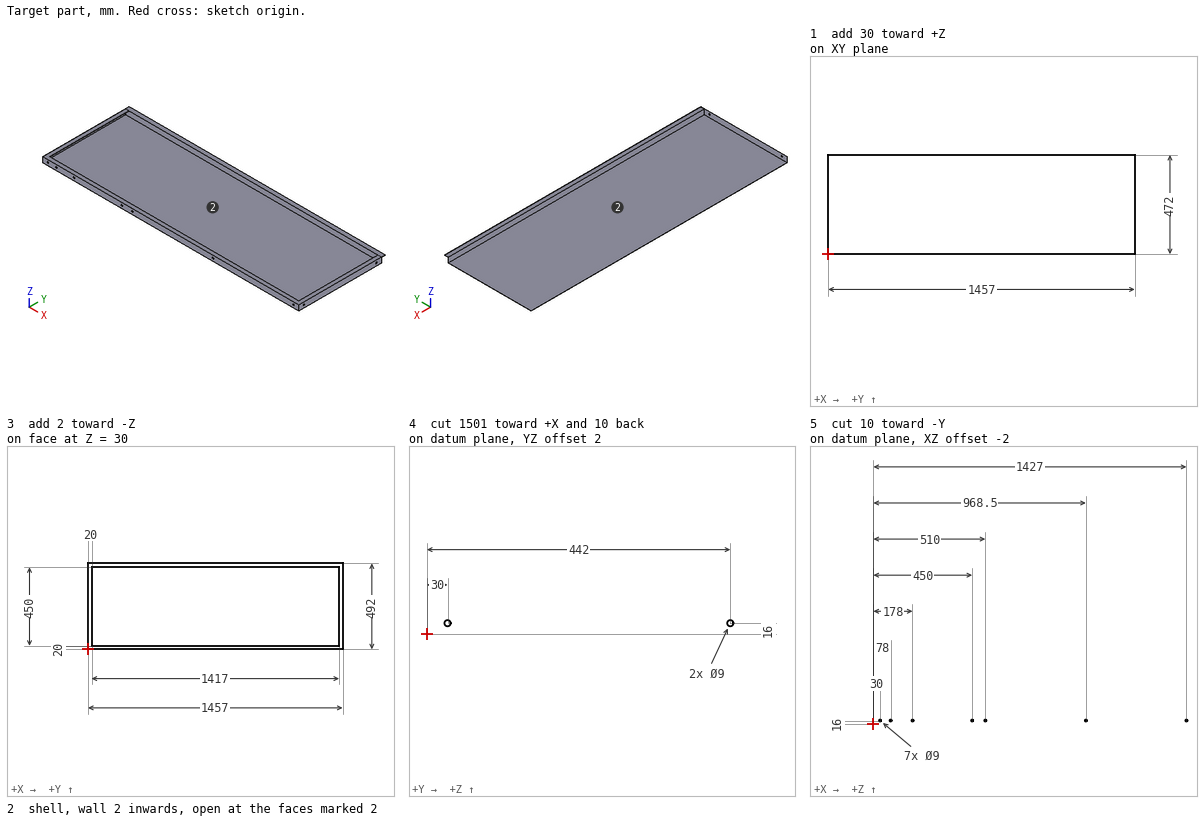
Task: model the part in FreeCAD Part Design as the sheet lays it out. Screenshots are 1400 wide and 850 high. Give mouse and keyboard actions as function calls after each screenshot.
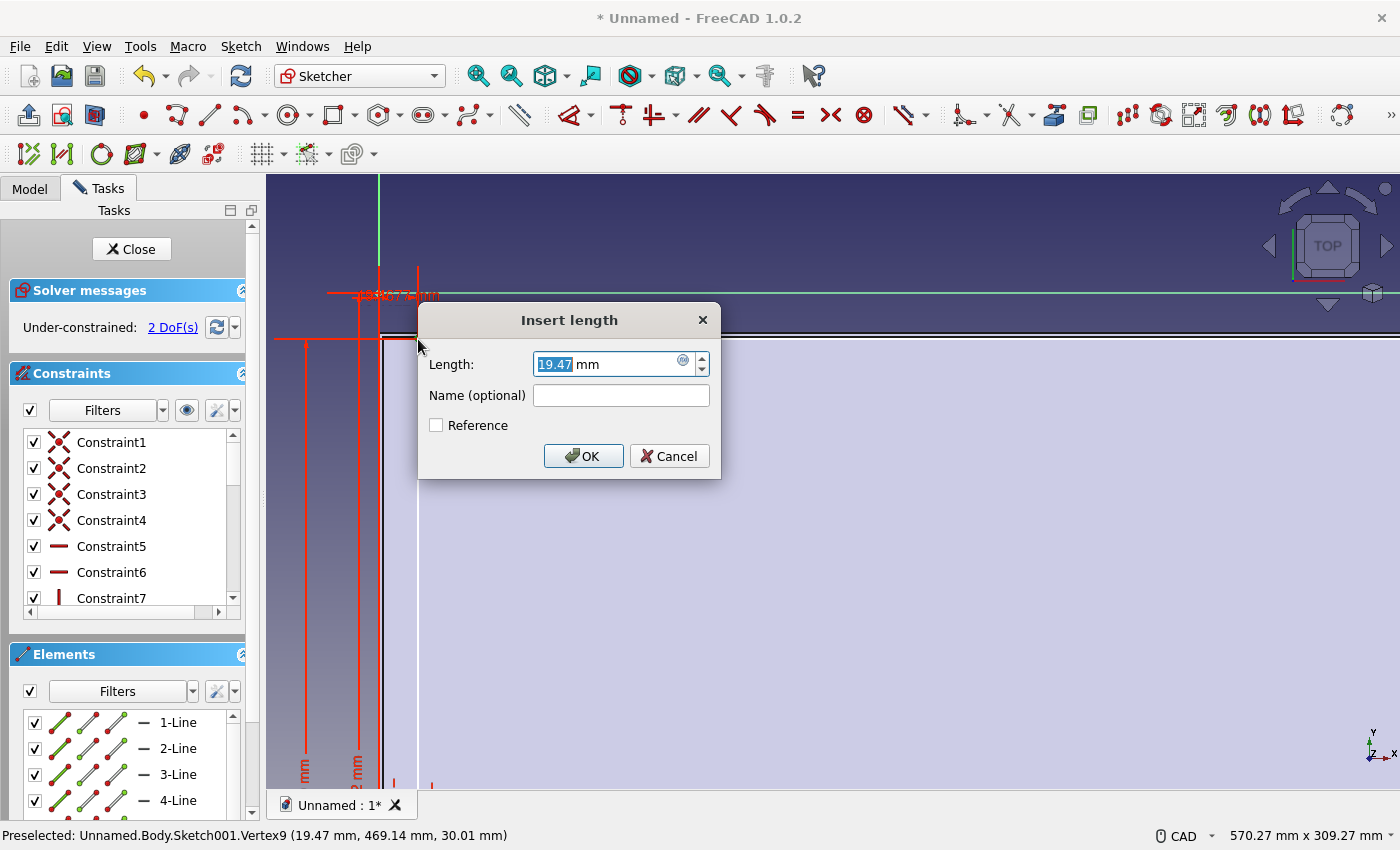
text(20)
key(Return)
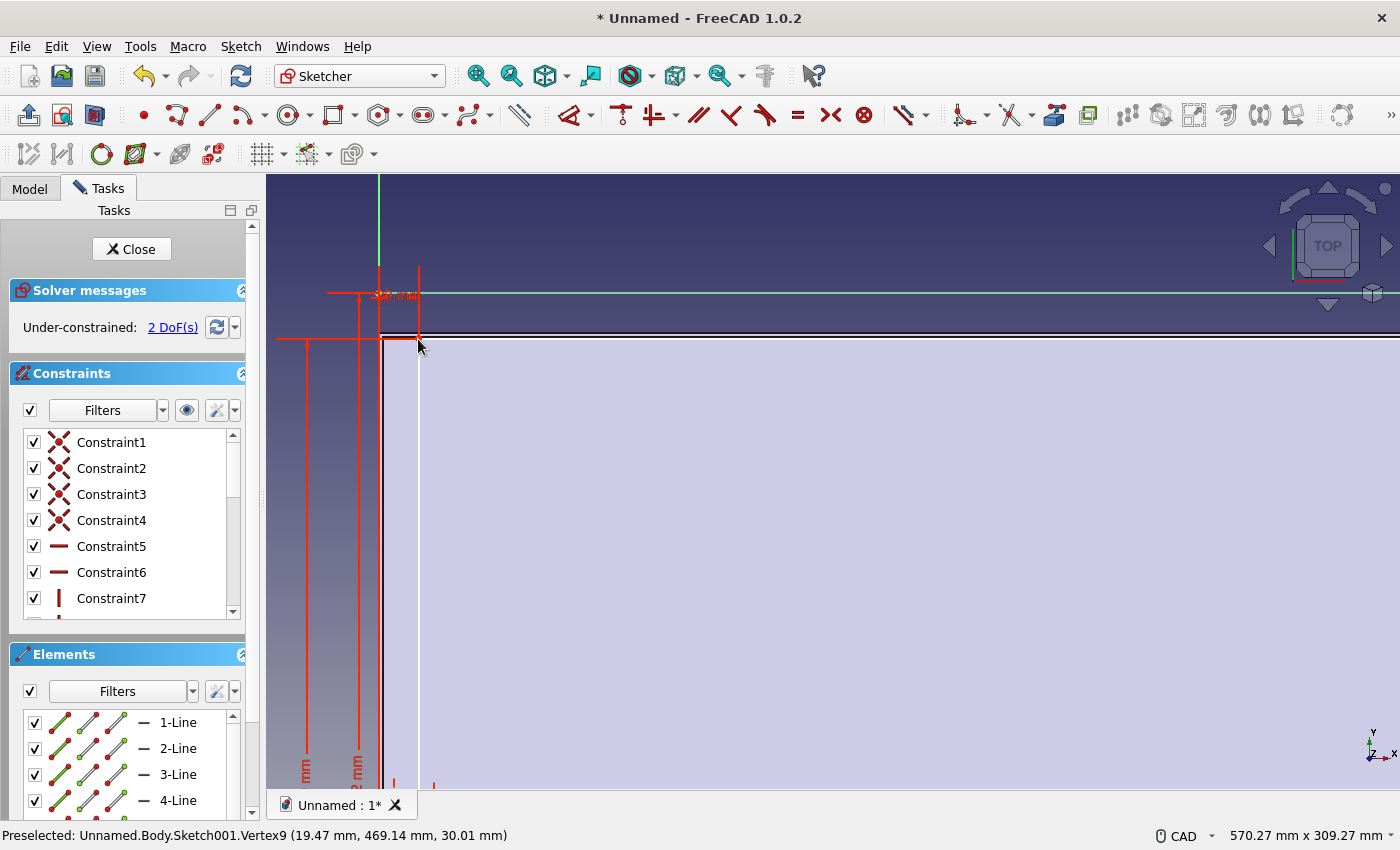
scroll(417, 383, down, 7)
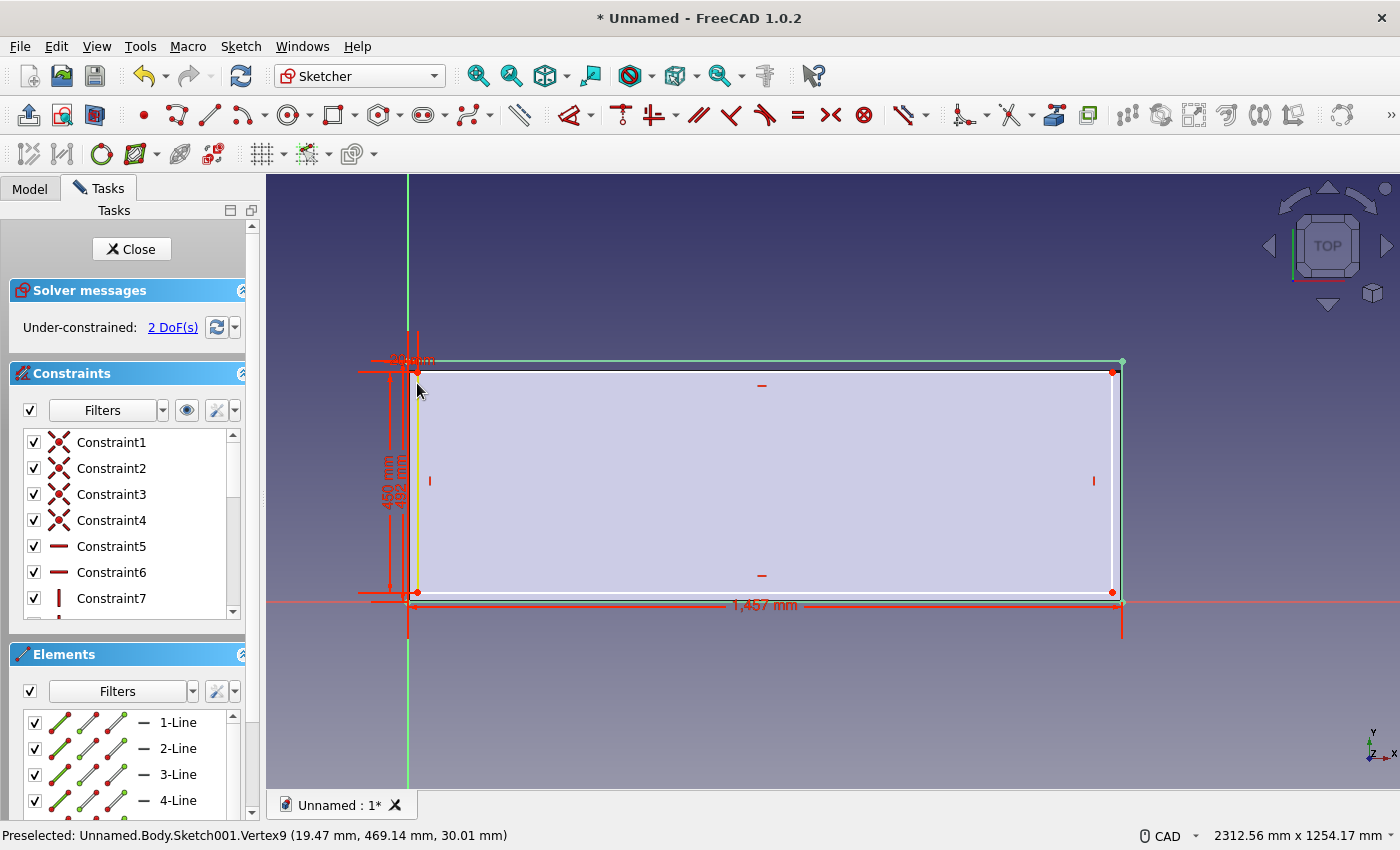
scroll(418, 593, up, 7)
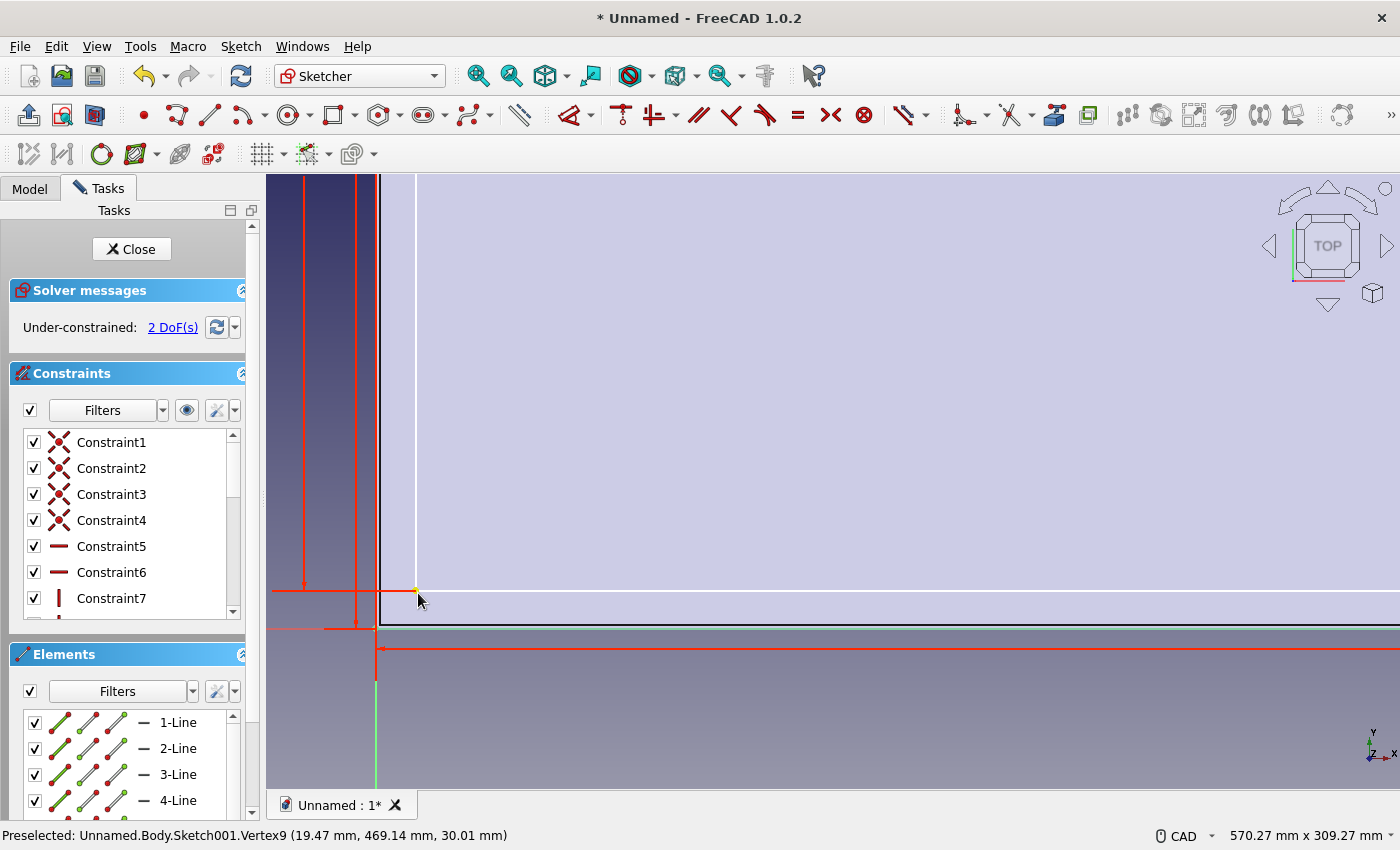
click(416, 591)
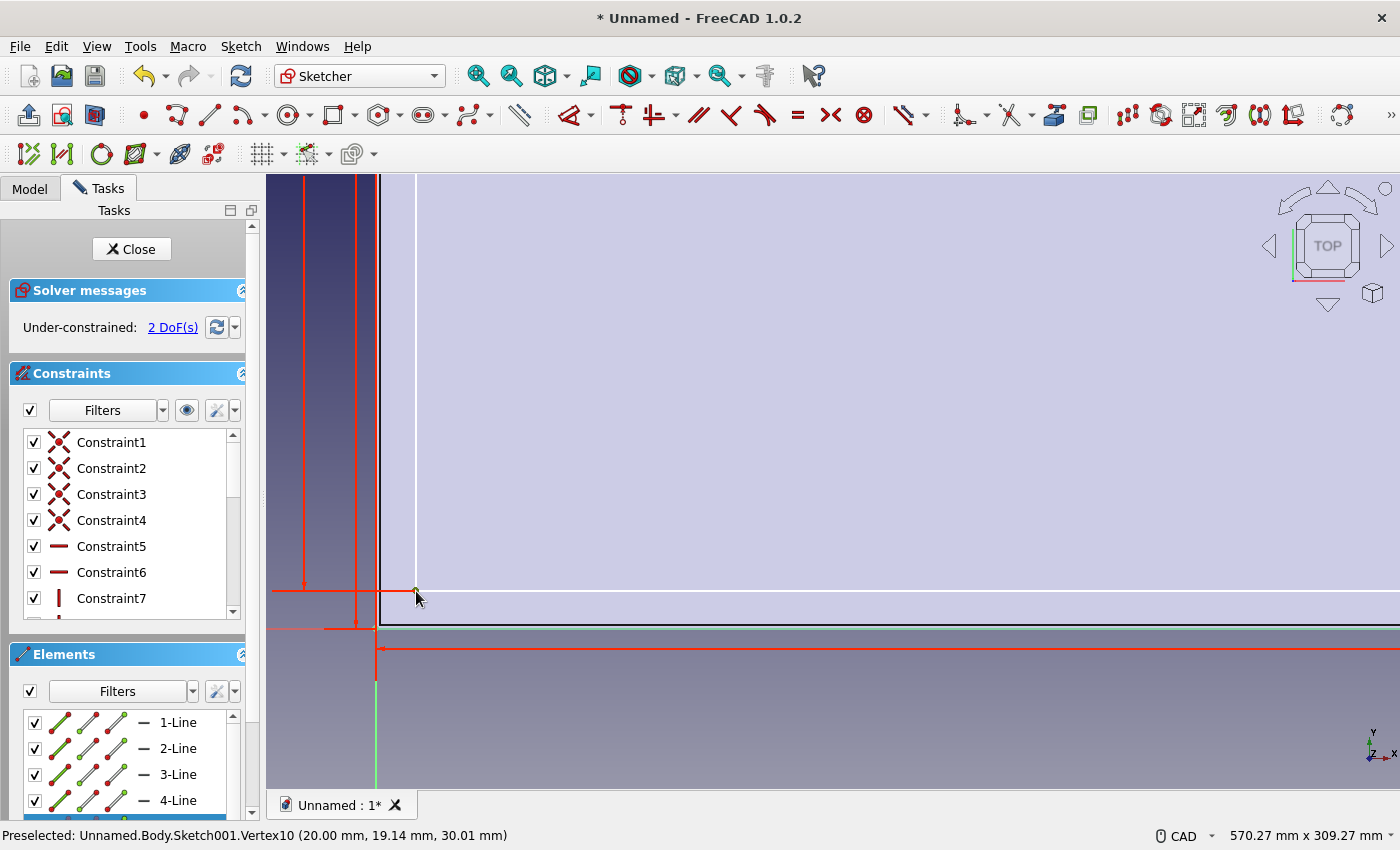
key(i)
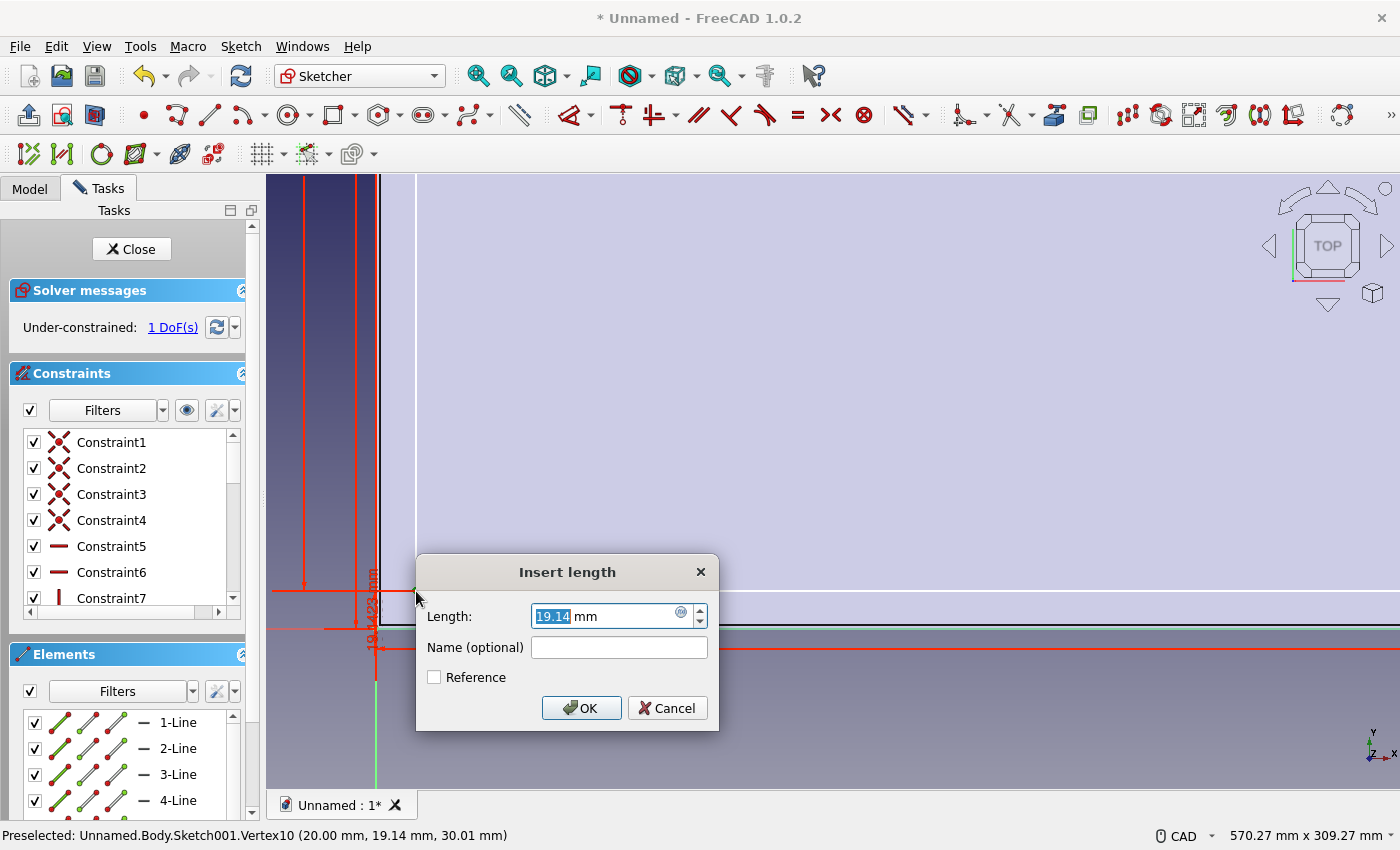
text(20)
key(Return)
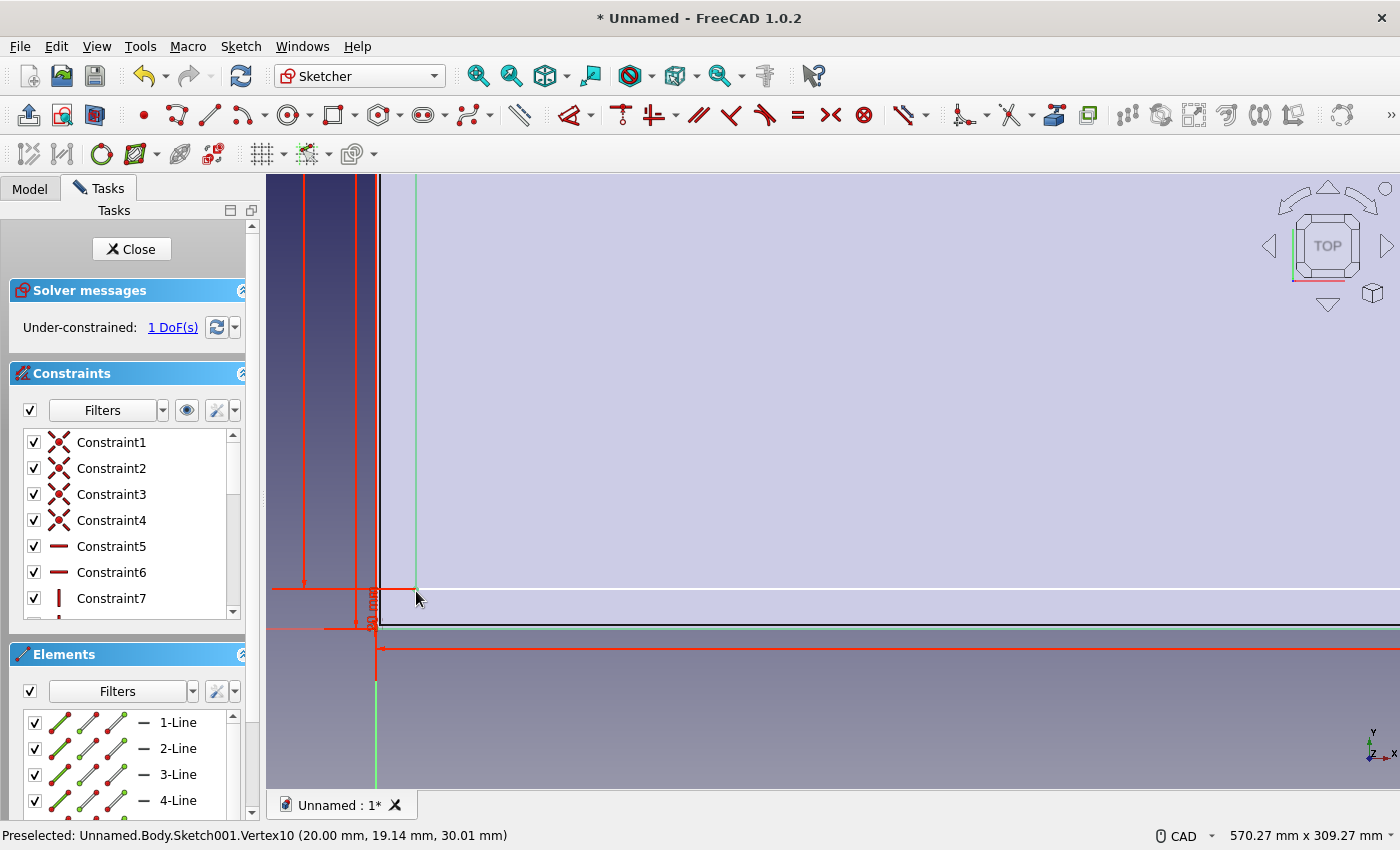
click(979, 589)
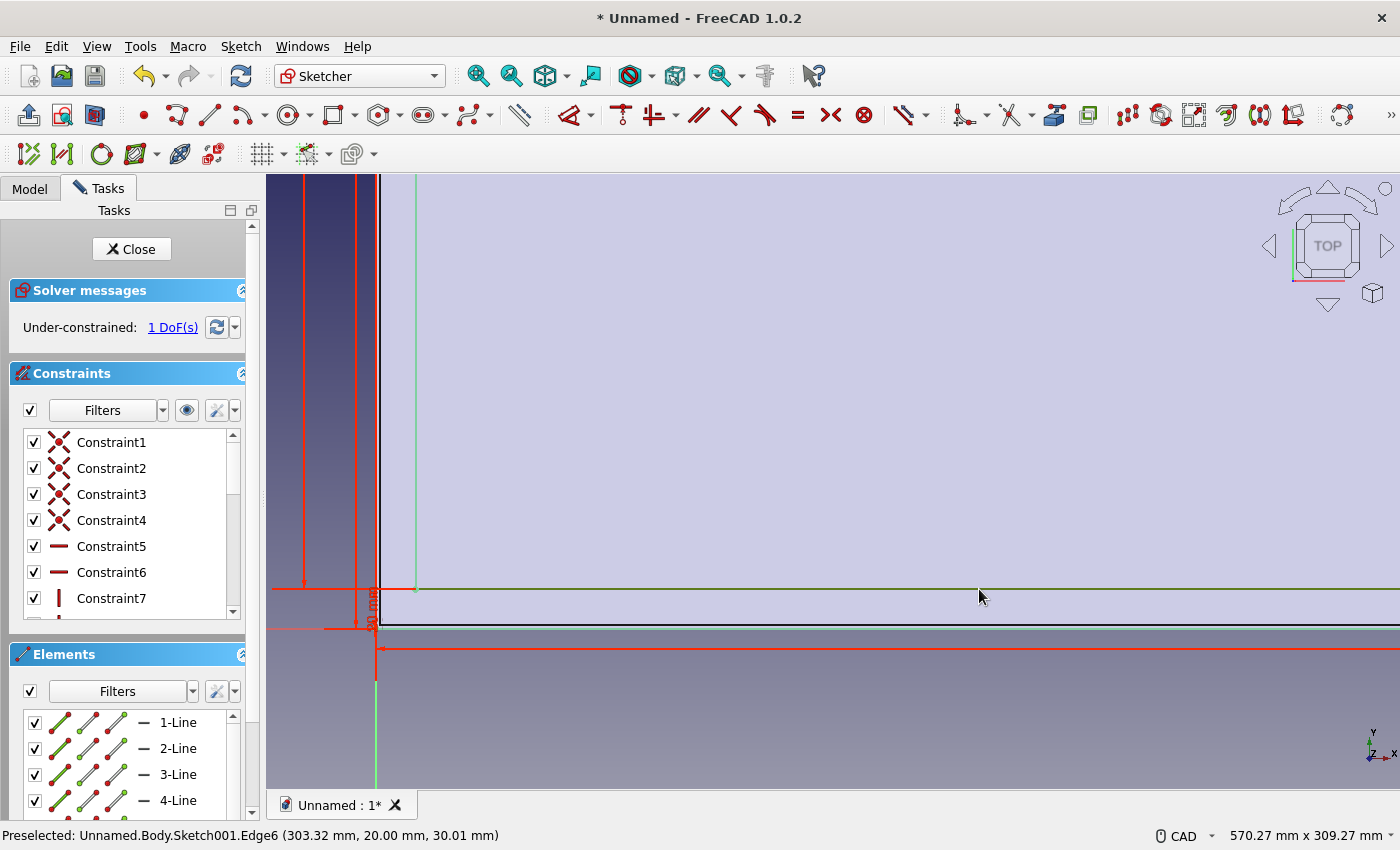
click(590, 116)